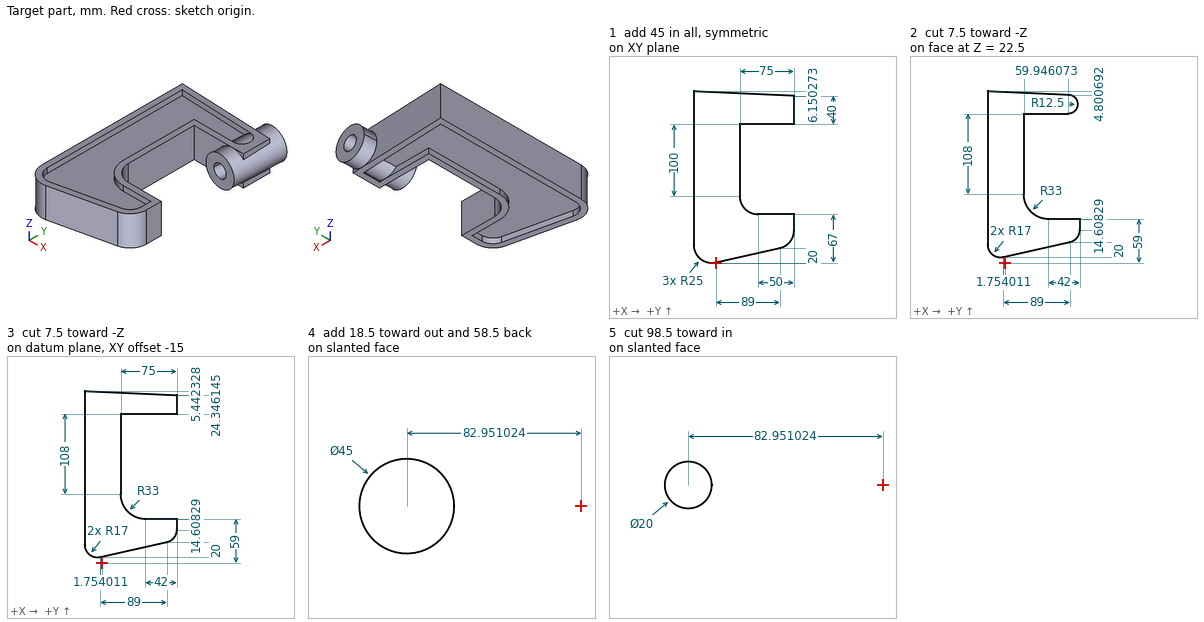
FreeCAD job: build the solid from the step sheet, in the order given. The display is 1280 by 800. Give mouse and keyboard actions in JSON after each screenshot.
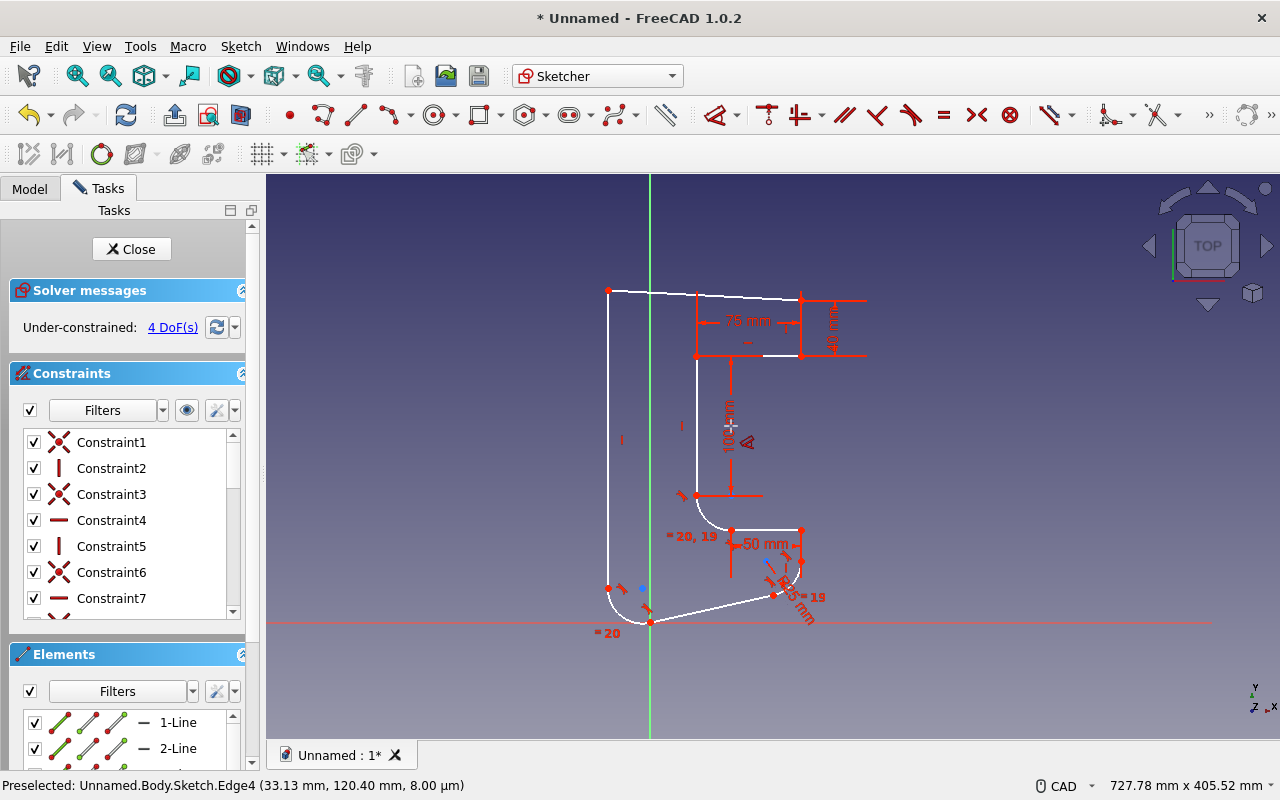
{"action": "left_click", "coordinate": [774, 595]}
{"action": "left_click", "coordinate": [712, 657]}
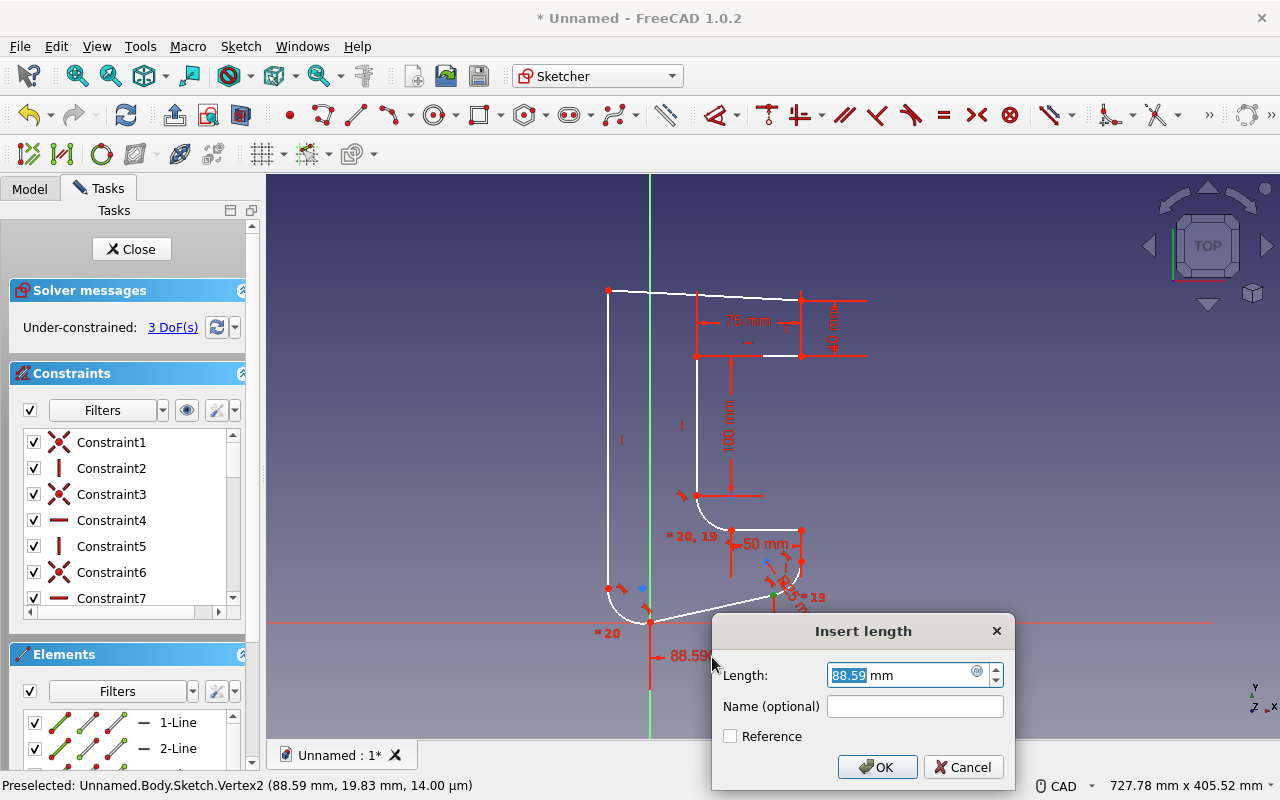
{"action": "type", "text": "89"}
{"action": "key", "text": "Return"}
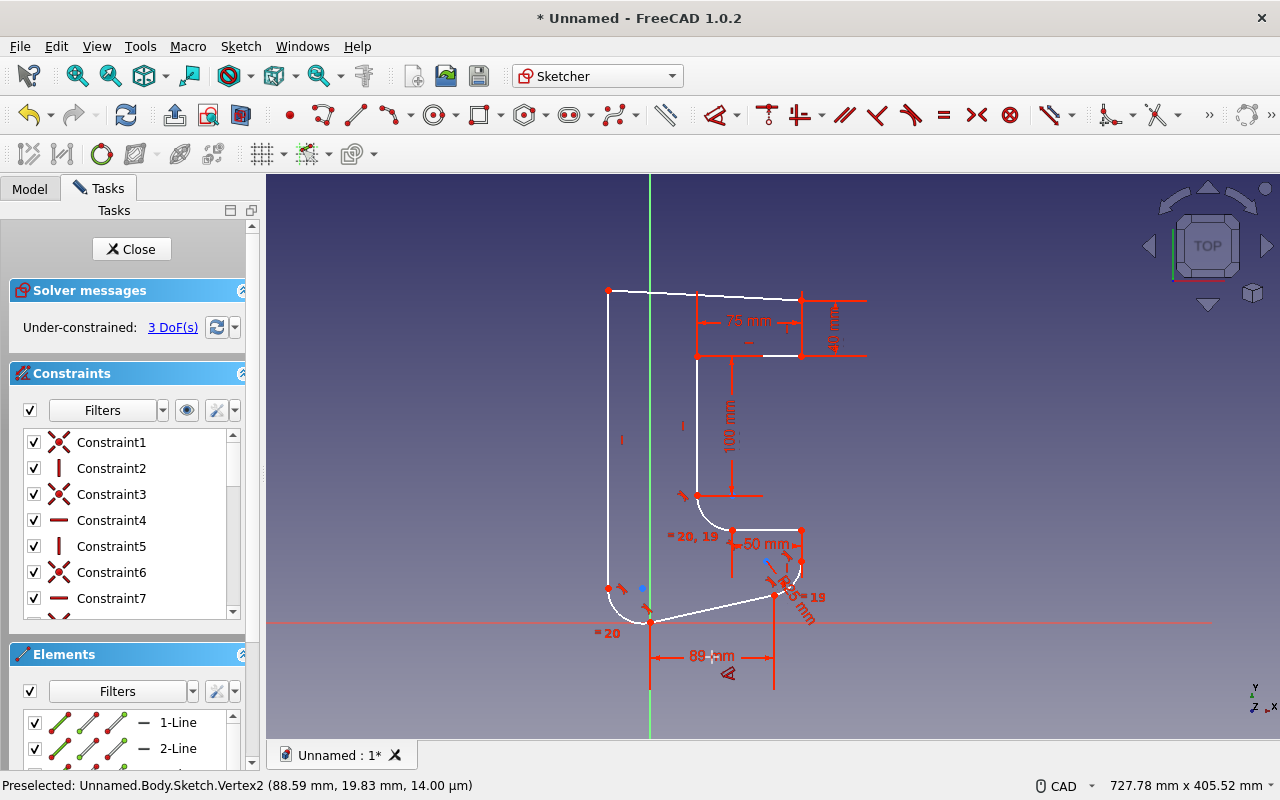
{"action": "scroll", "coordinate": [774, 595], "scroll_direction": "up", "scroll_amount": 2}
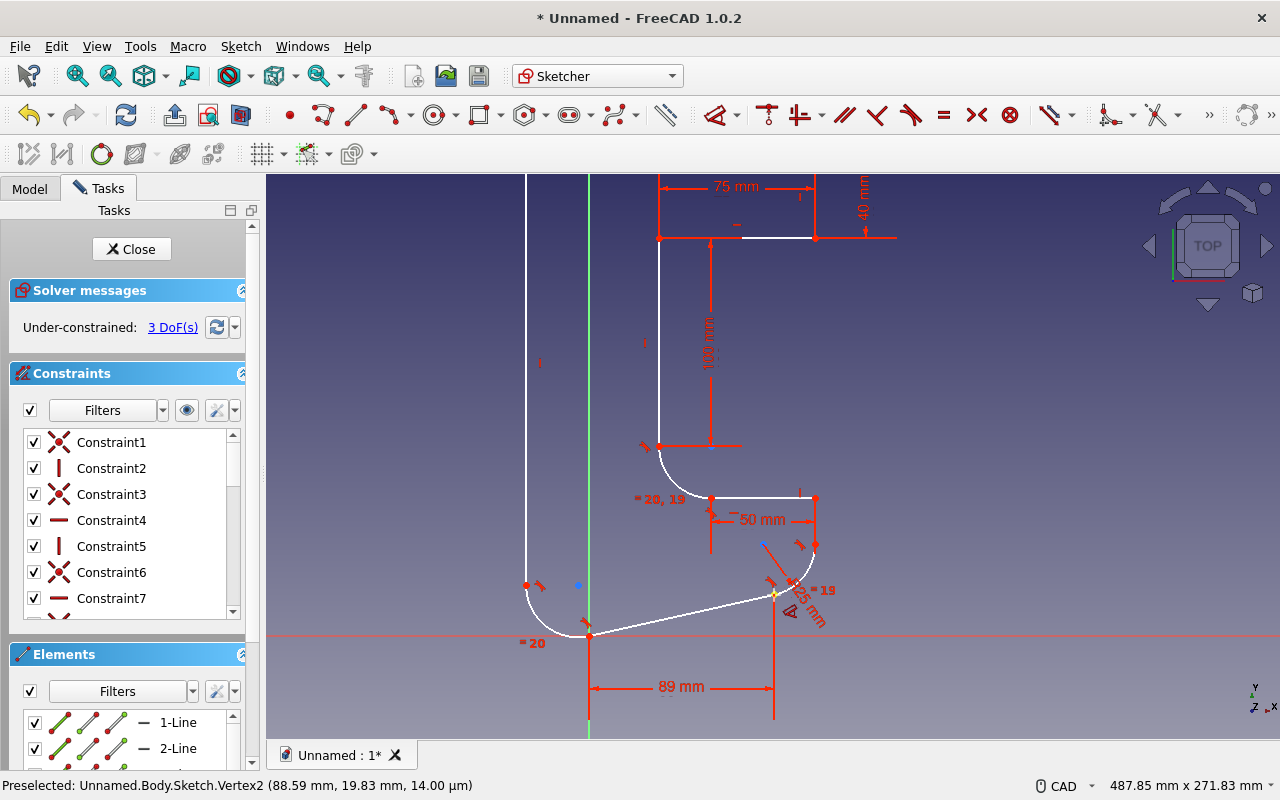
{"action": "left_click", "coordinate": [774, 595]}
{"action": "left_click", "coordinate": [555, 615]}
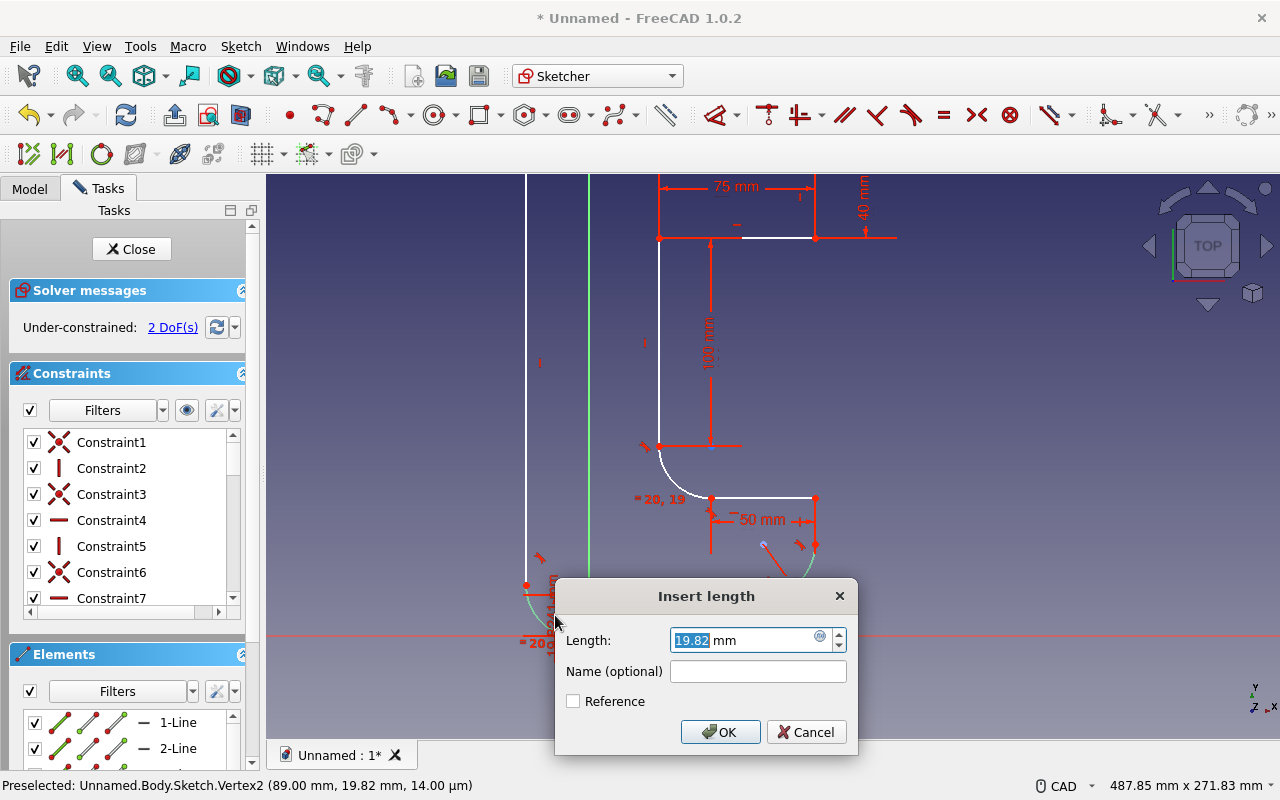
{"action": "type", "text": "20"}
{"action": "key", "text": "Return"}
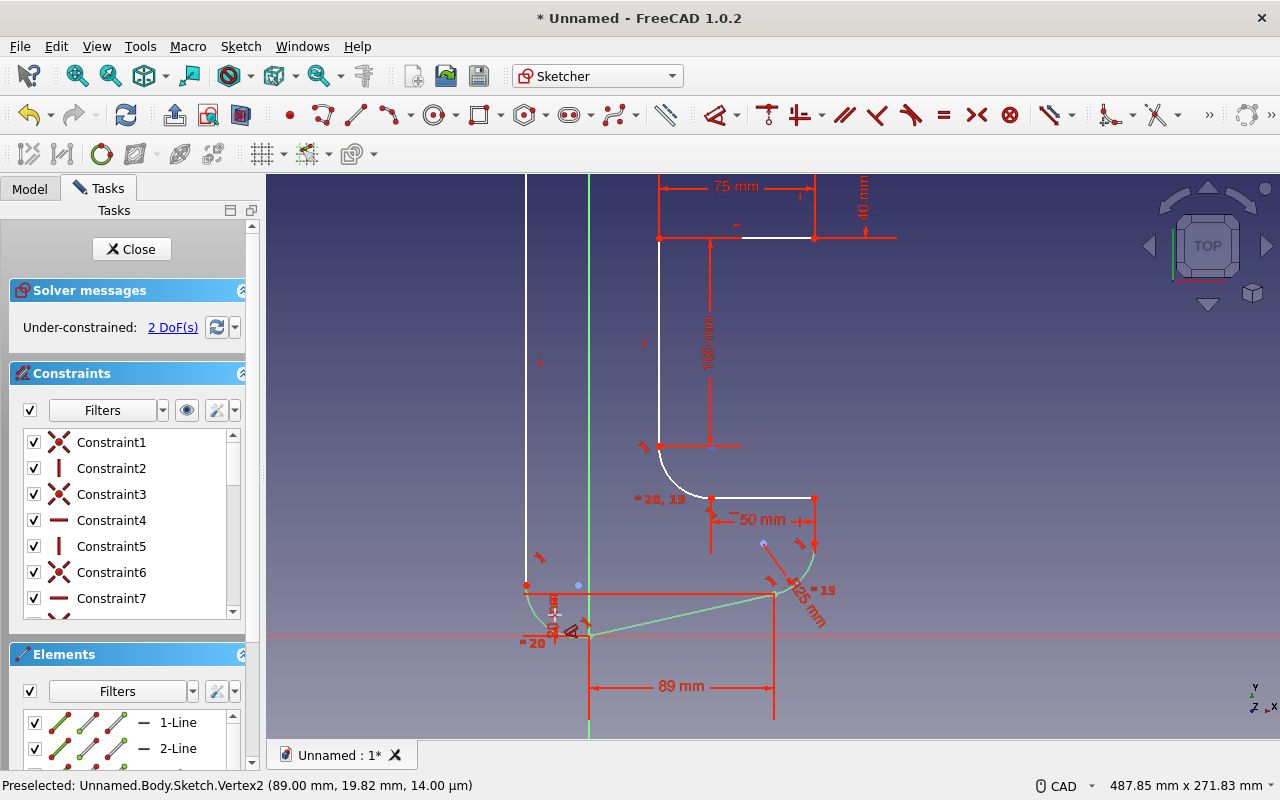
{"action": "left_click", "coordinate": [815, 498]}
{"action": "left_click", "coordinate": [849, 567]}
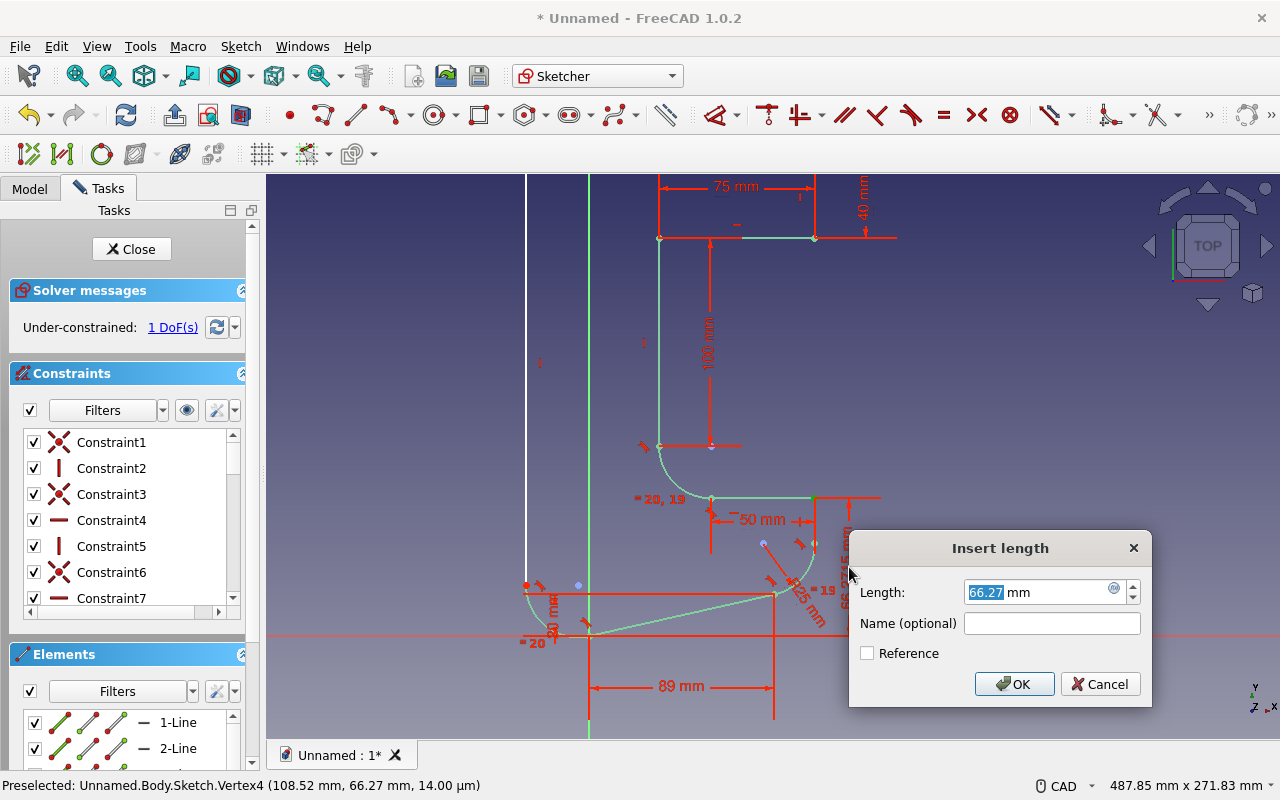
{"action": "type", "text": "67"}
{"action": "key", "text": "Return"}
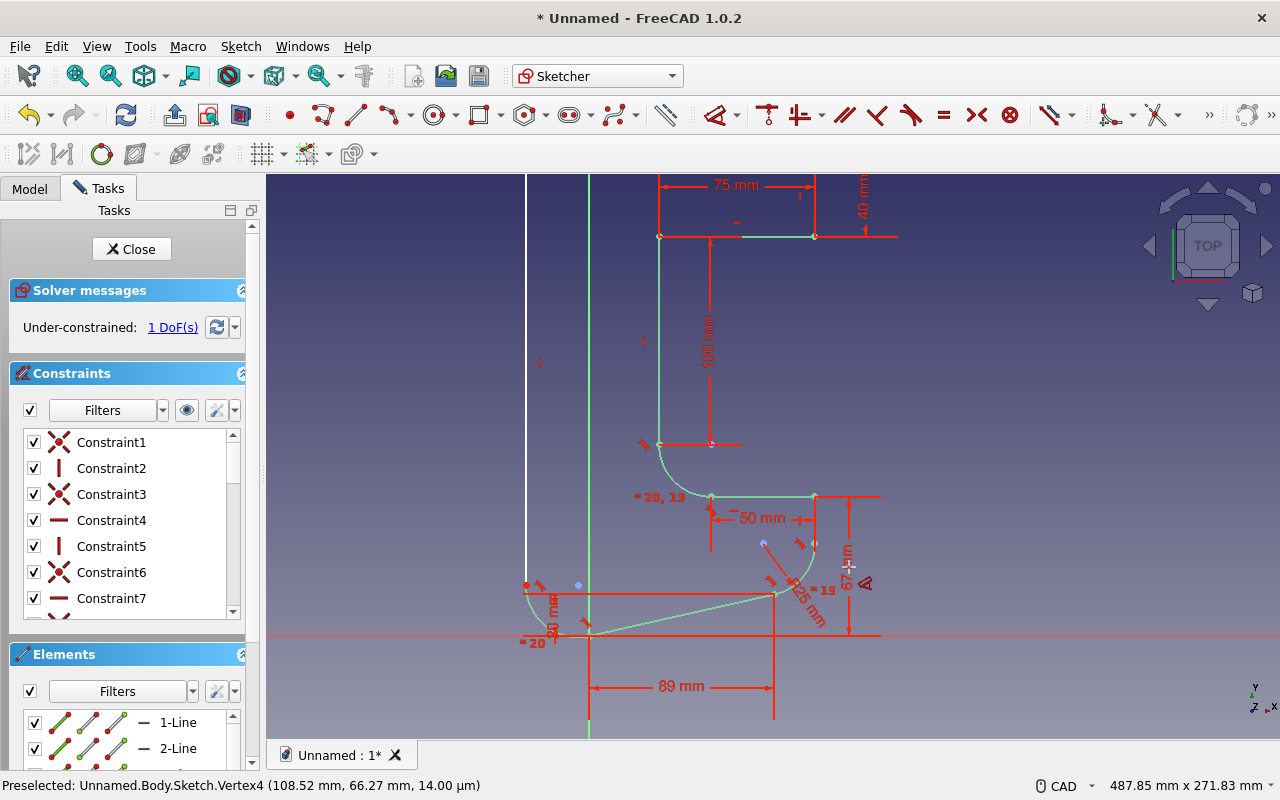
{"action": "scroll", "coordinate": [774, 595], "scroll_direction": "down", "scroll_amount": 2}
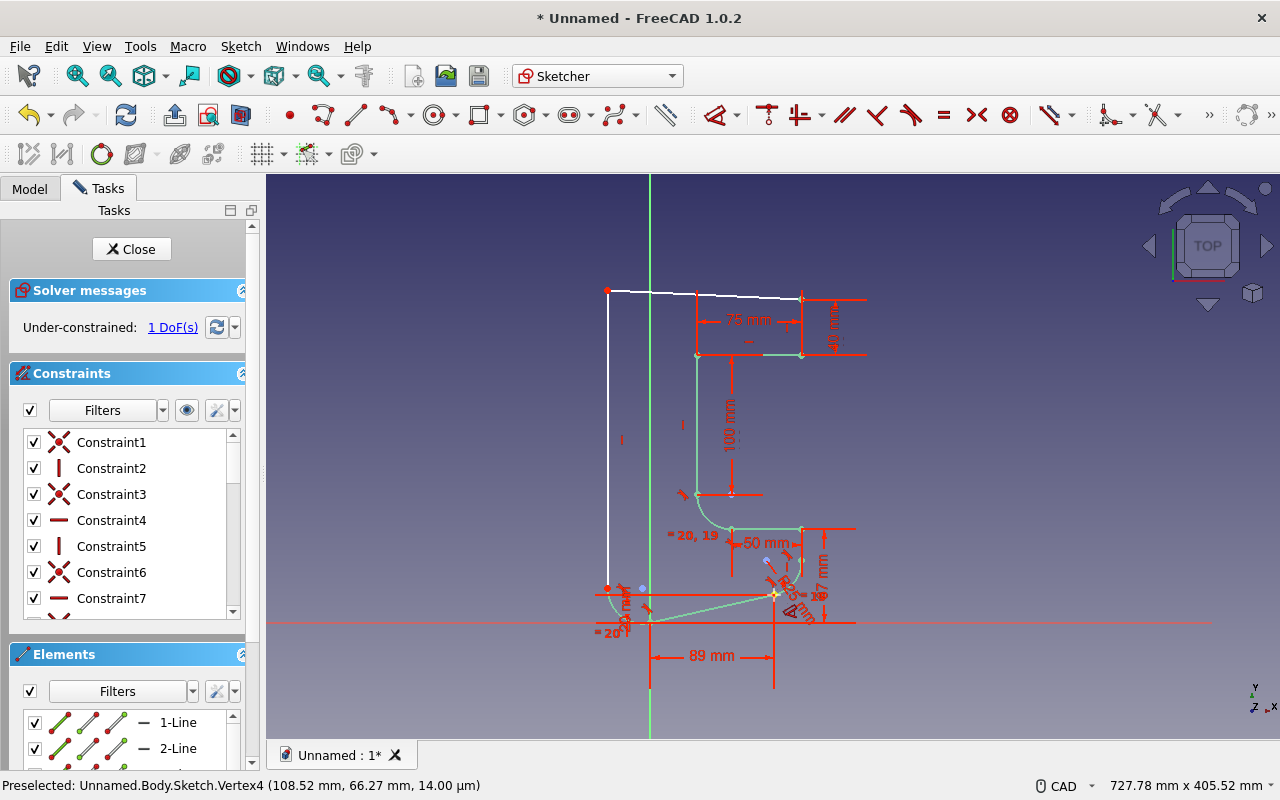
{"action": "scroll", "coordinate": [744, 297], "scroll_direction": "up", "scroll_amount": 8}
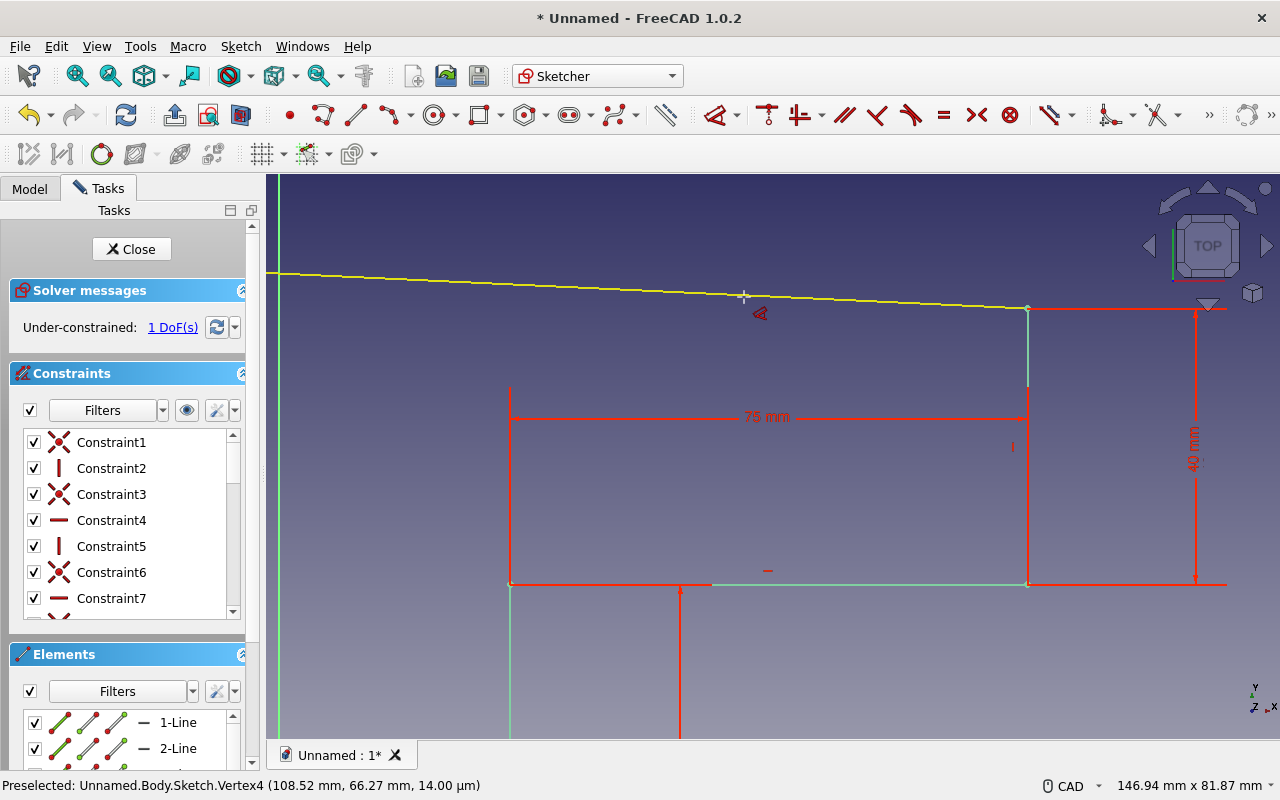
{"action": "left_click", "coordinate": [740, 295]}
{"action": "left_click", "coordinate": [1062, 286]}